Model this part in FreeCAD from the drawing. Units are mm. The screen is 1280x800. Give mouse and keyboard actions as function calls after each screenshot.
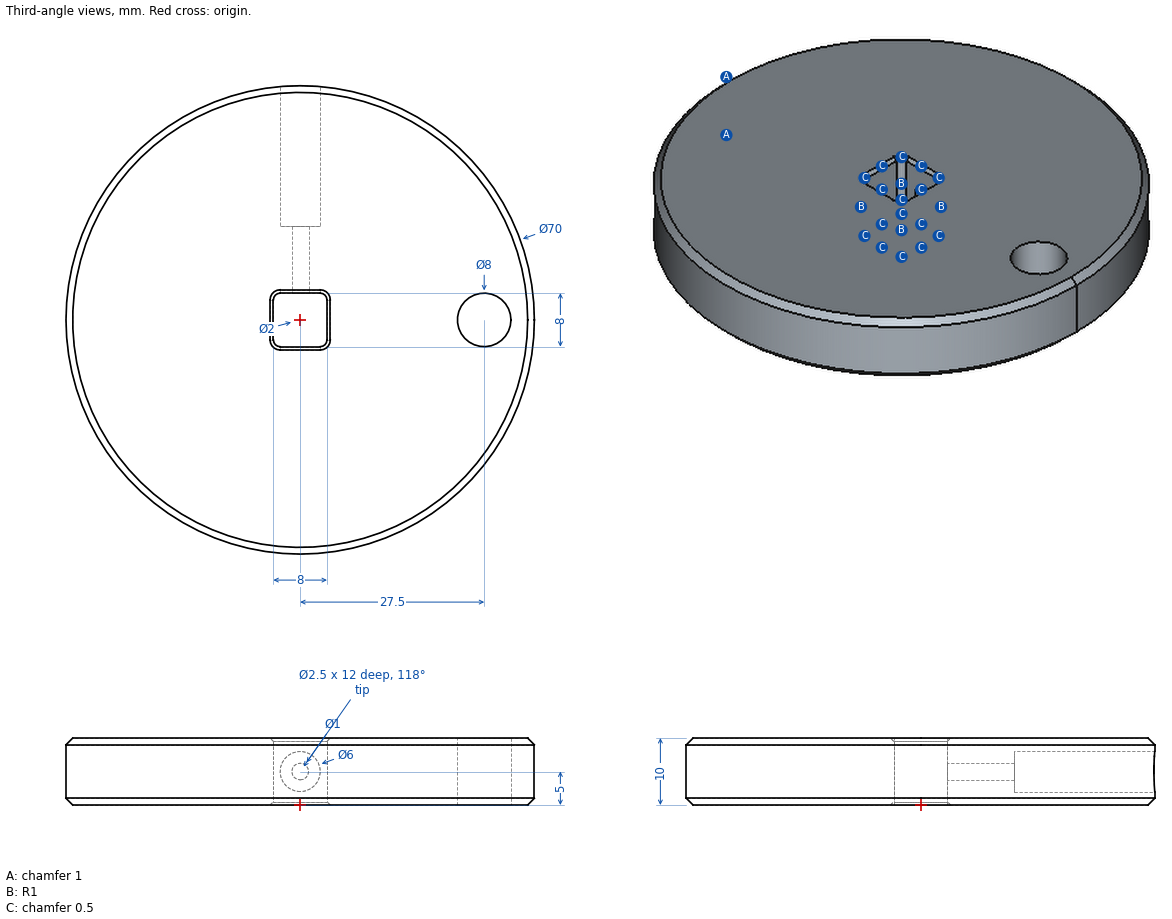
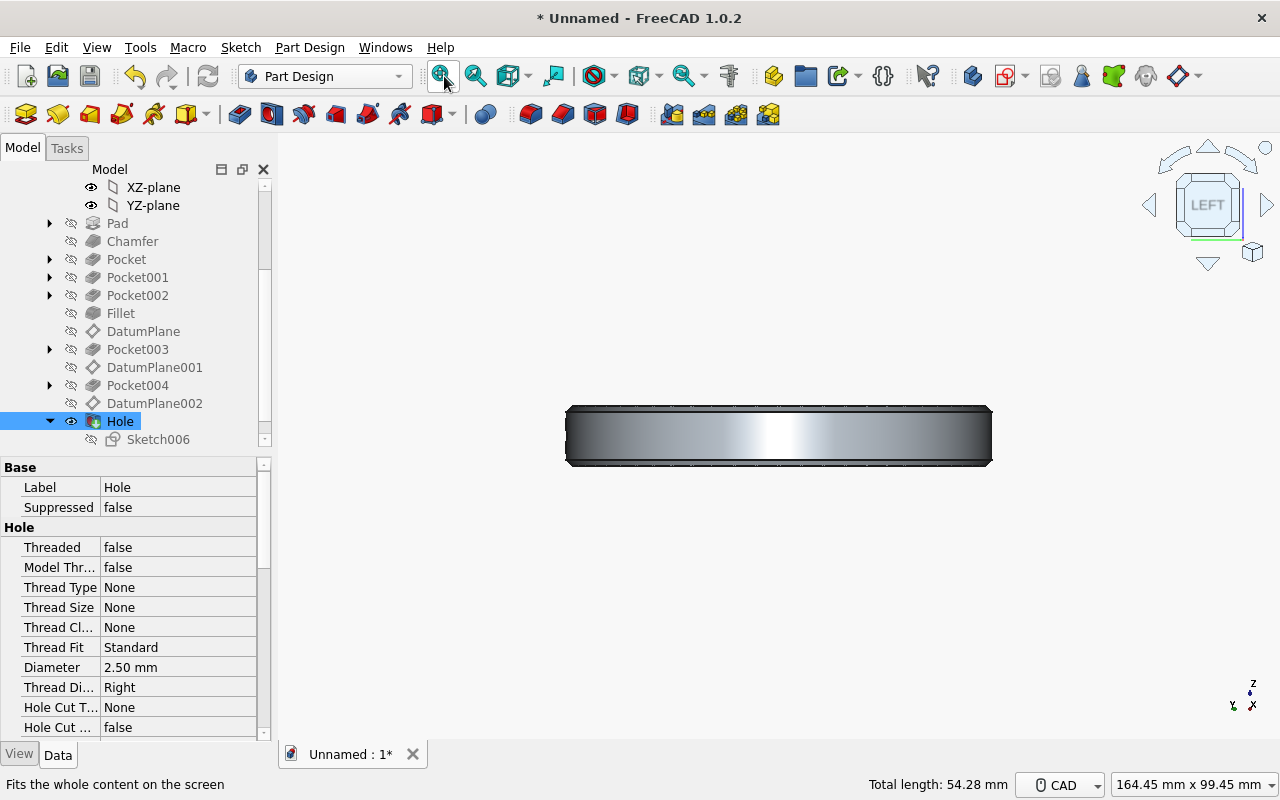
key(v)
key(3)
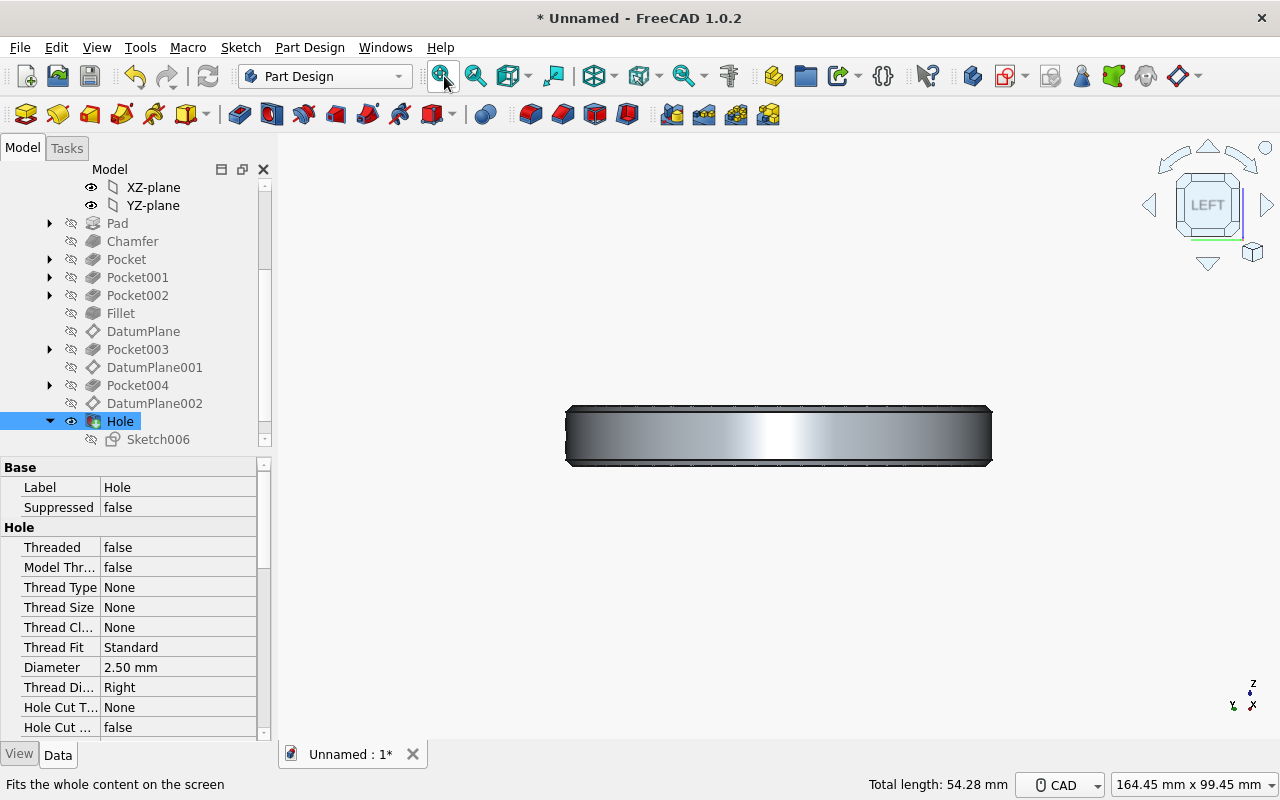
key(0)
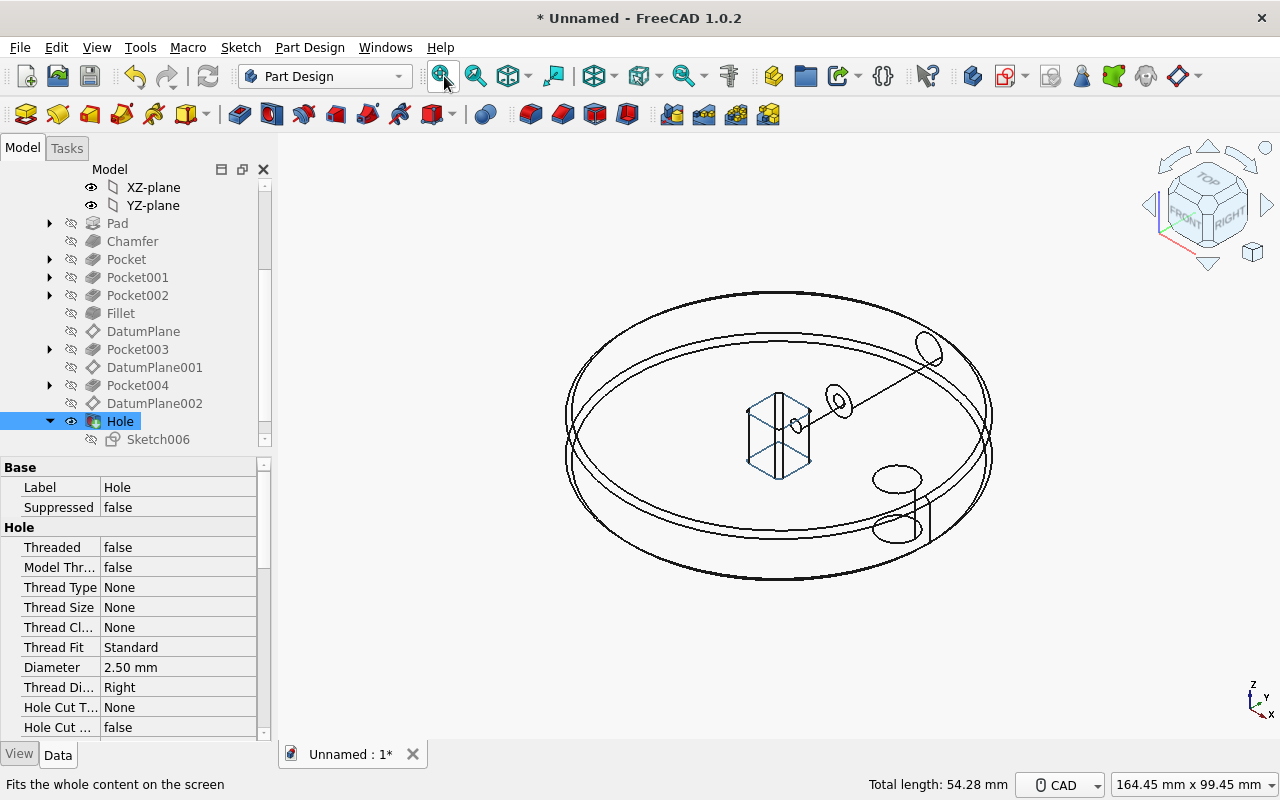
click(779, 429, ctrl)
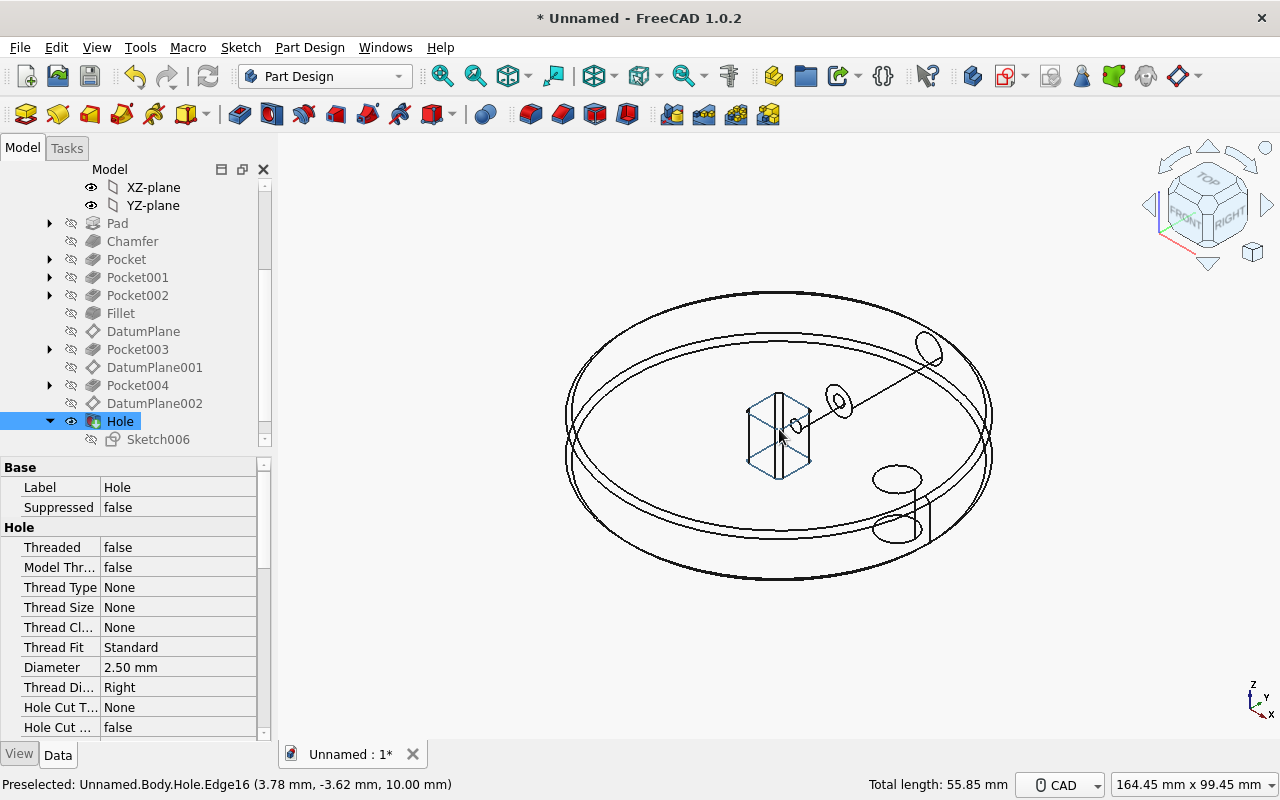
scroll(747, 410, up, 8)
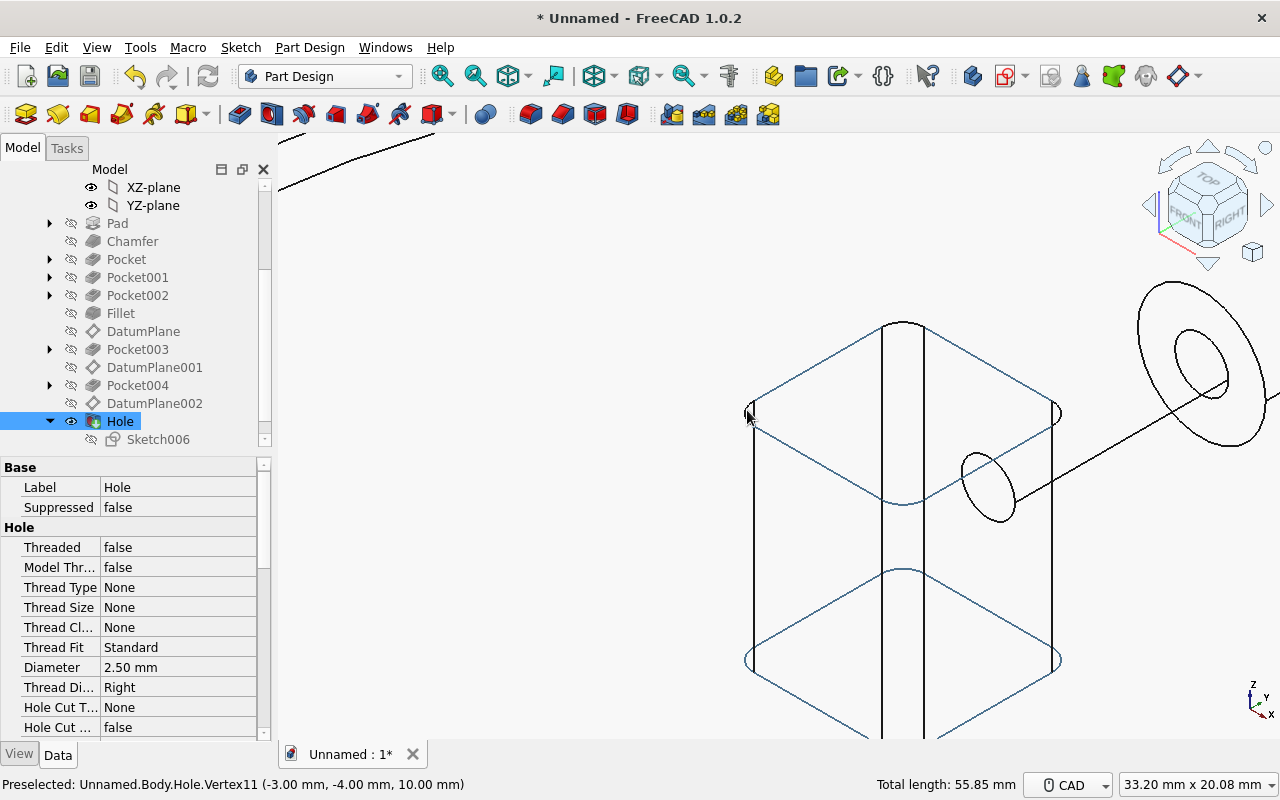
click(745, 413, ctrl)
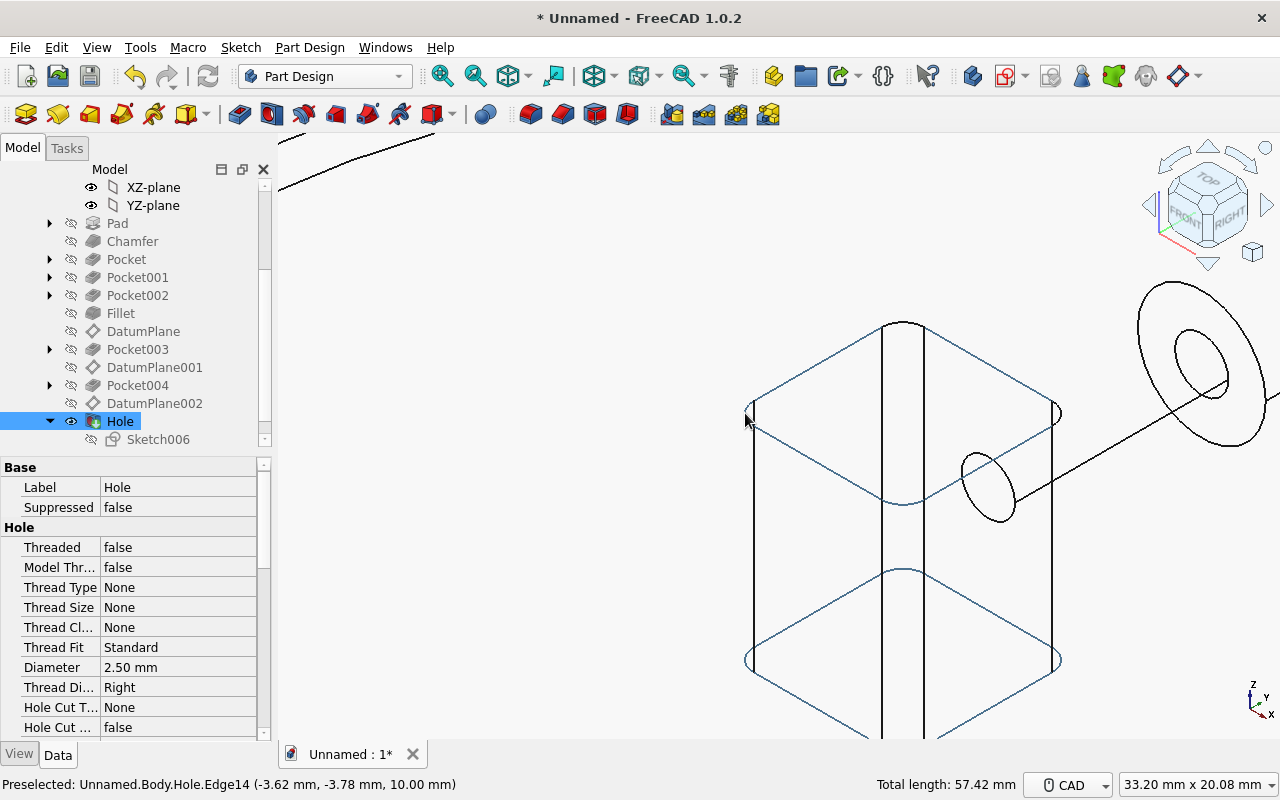
click(1061, 413, ctrl)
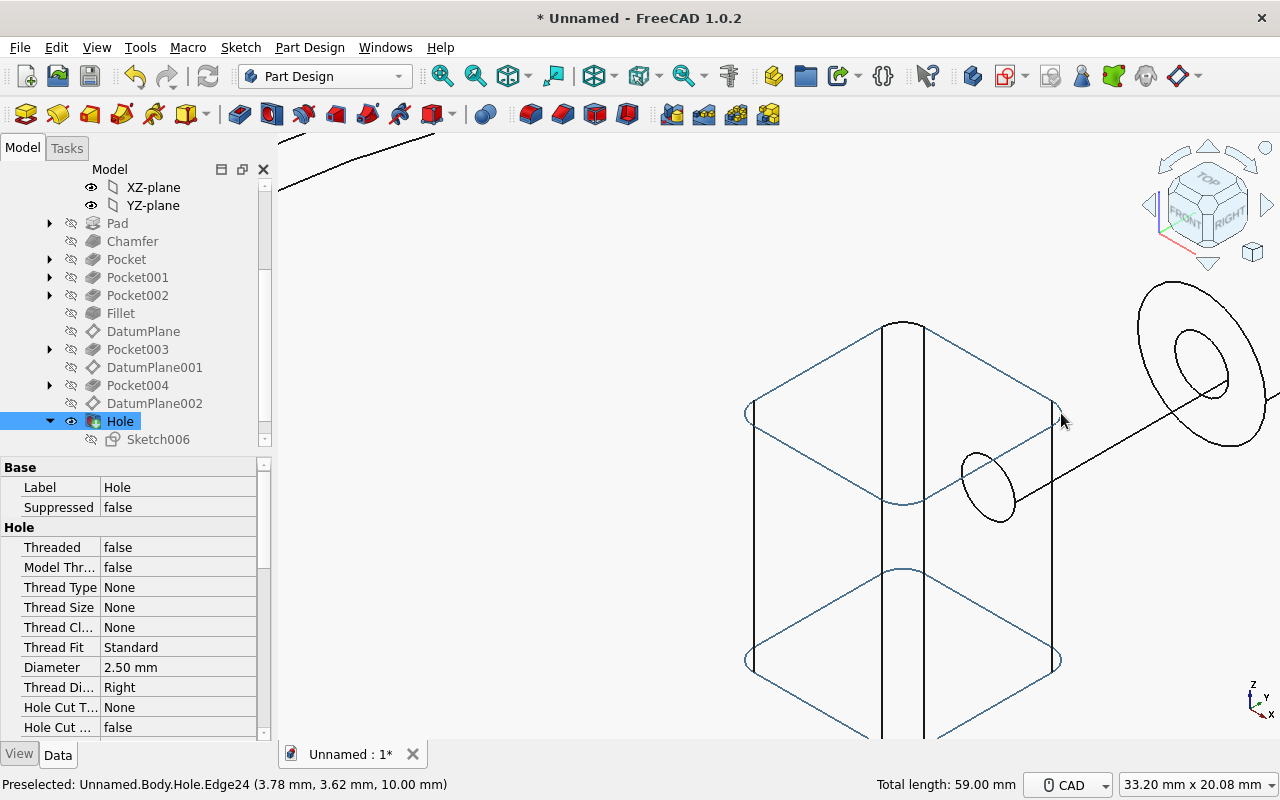
click(903, 321, ctrl)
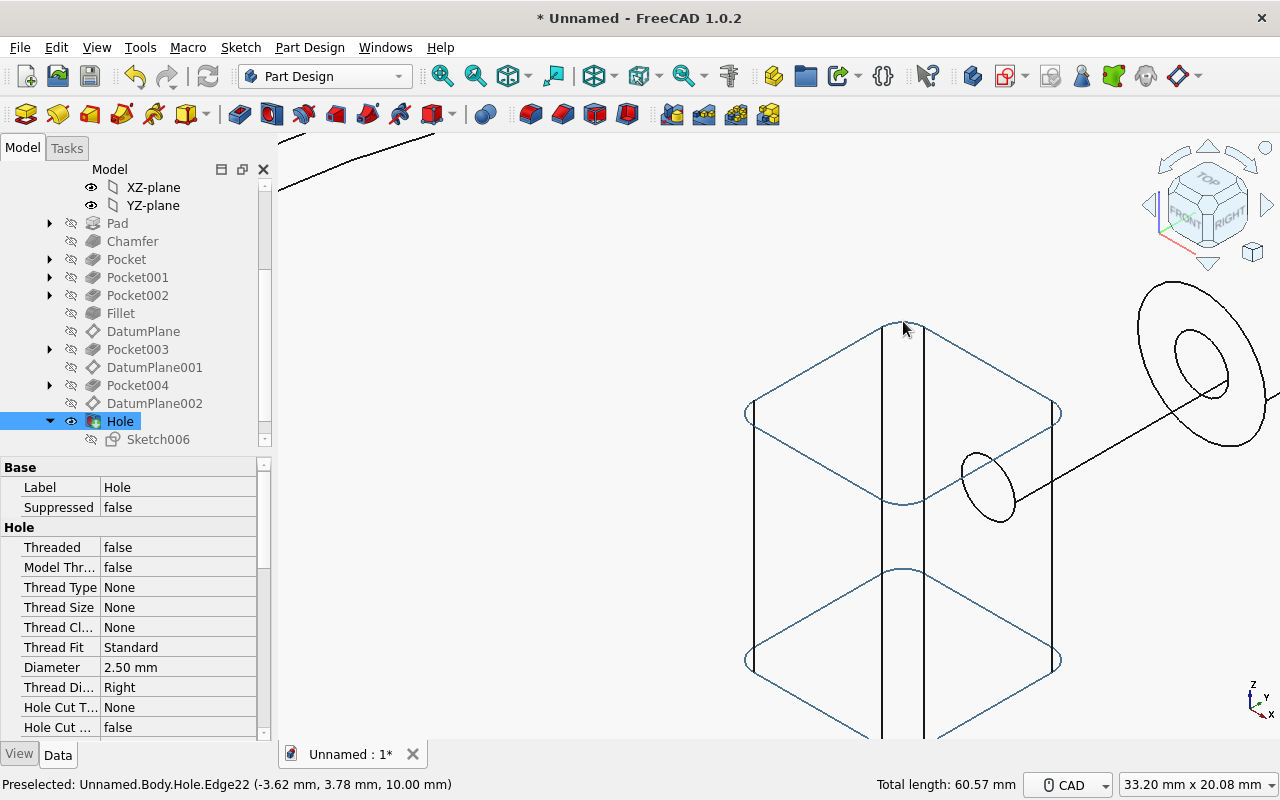
key(v)
key(1)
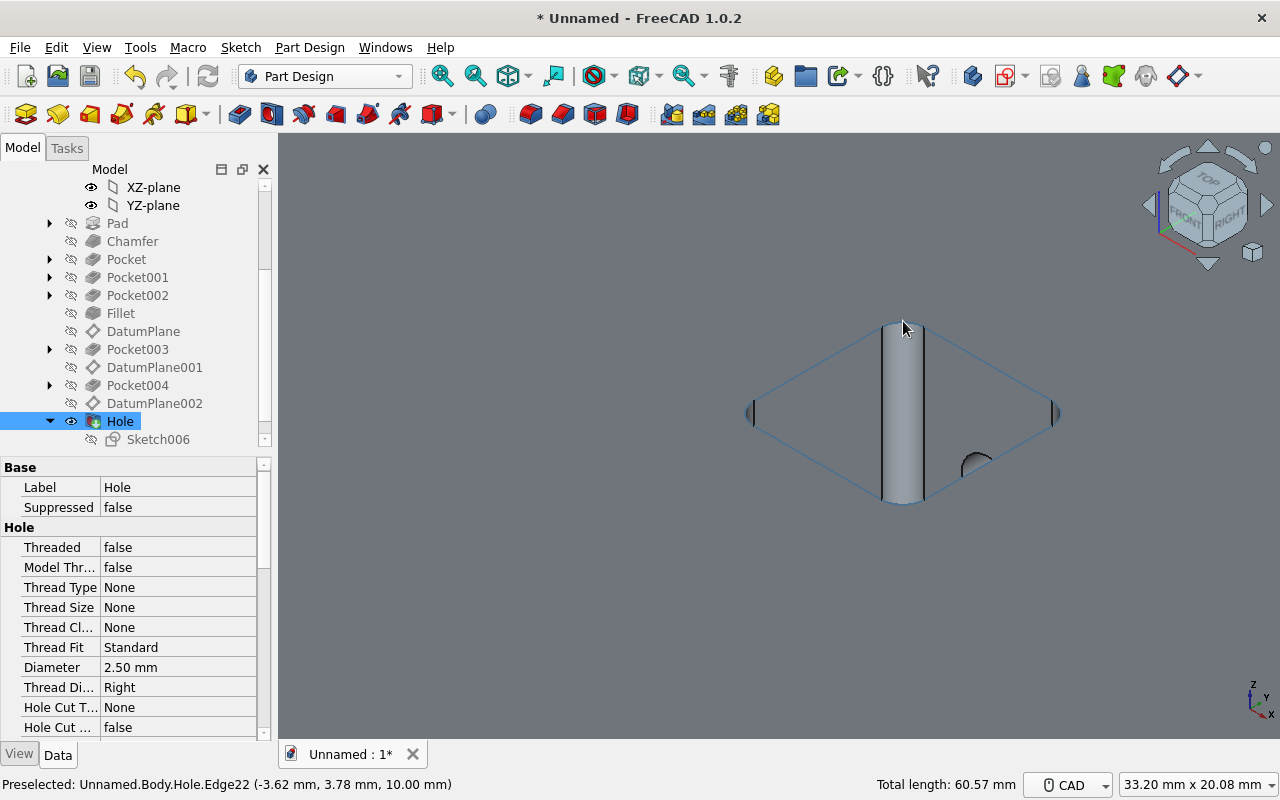
click(564, 114)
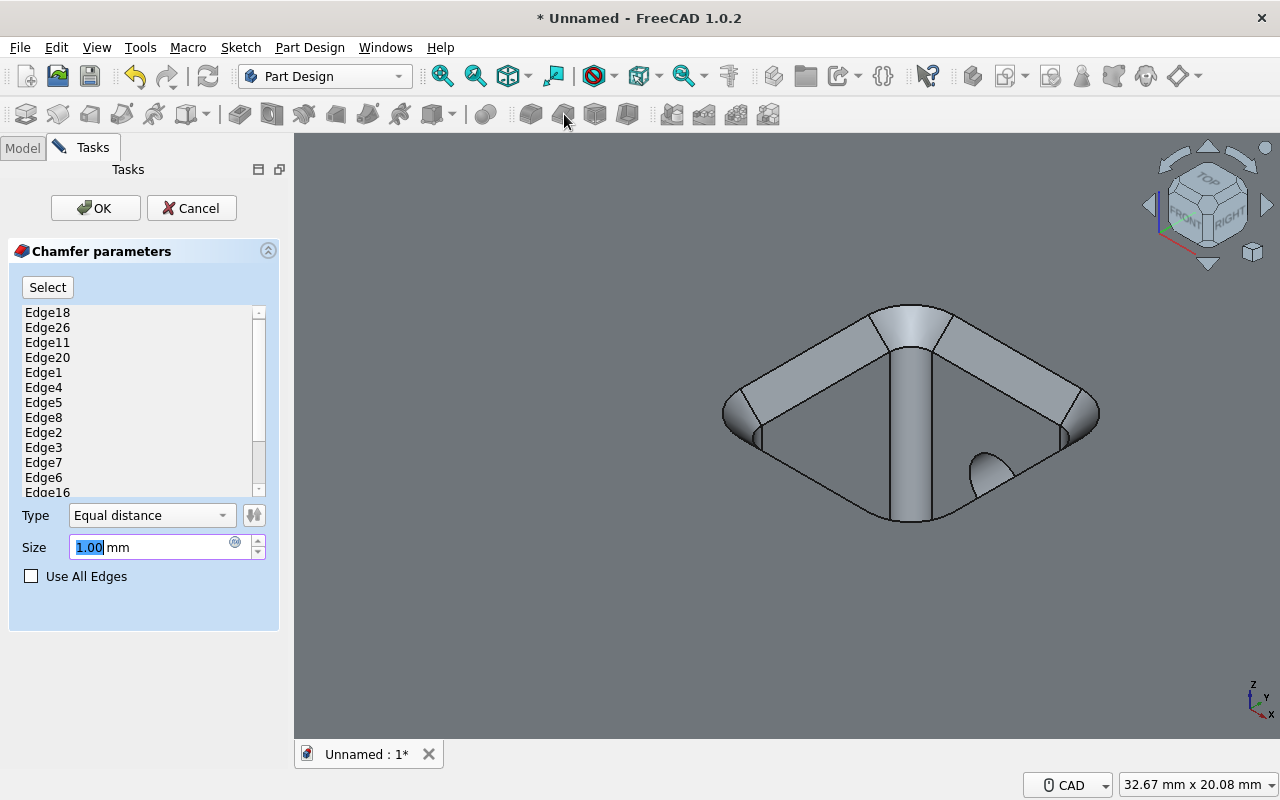
text(0.5)
key(Tab)